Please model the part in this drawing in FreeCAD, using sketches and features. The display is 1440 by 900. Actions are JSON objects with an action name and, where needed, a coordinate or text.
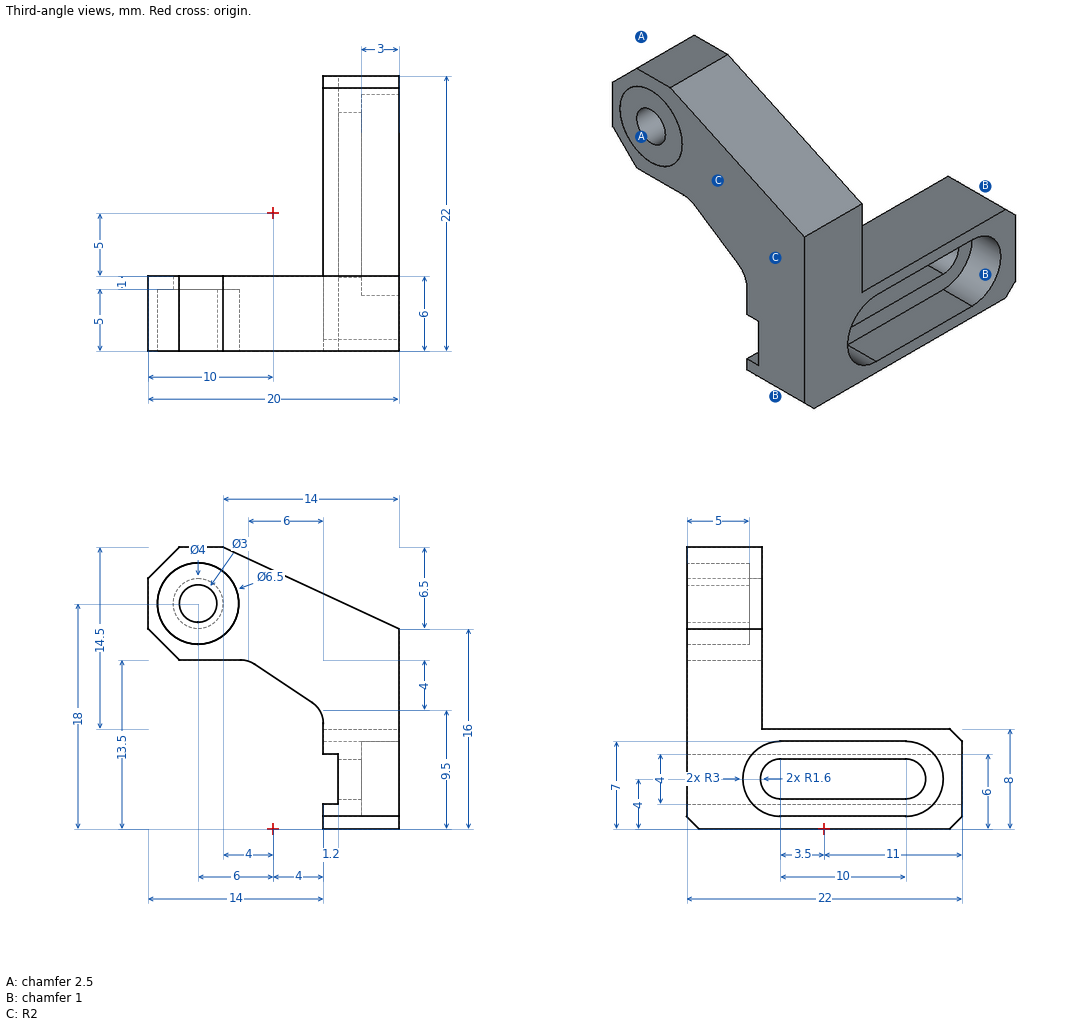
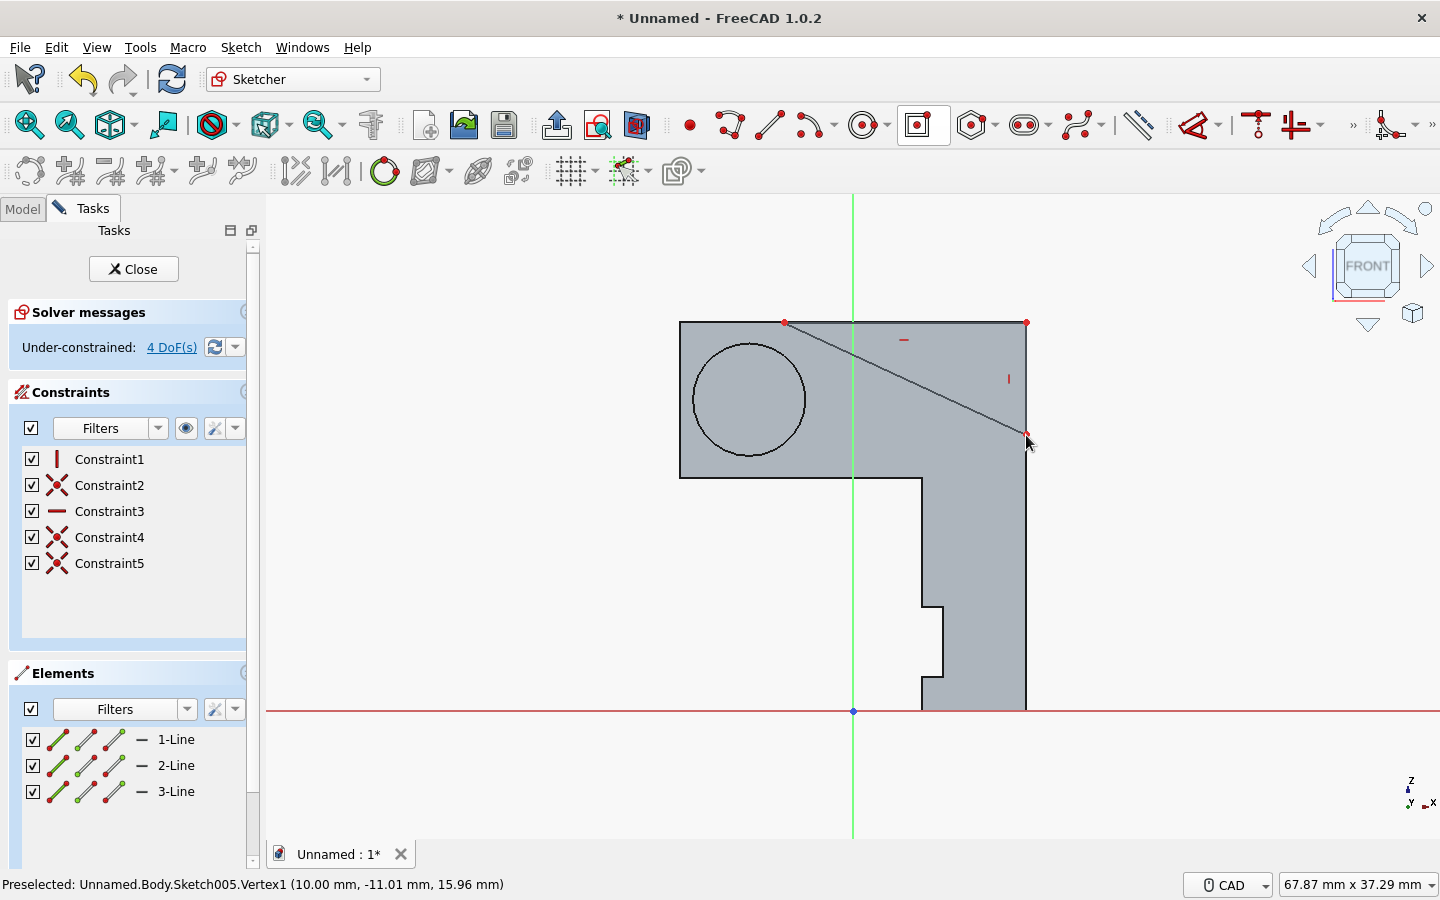
{"action": "left_click", "coordinate": [1194, 126]}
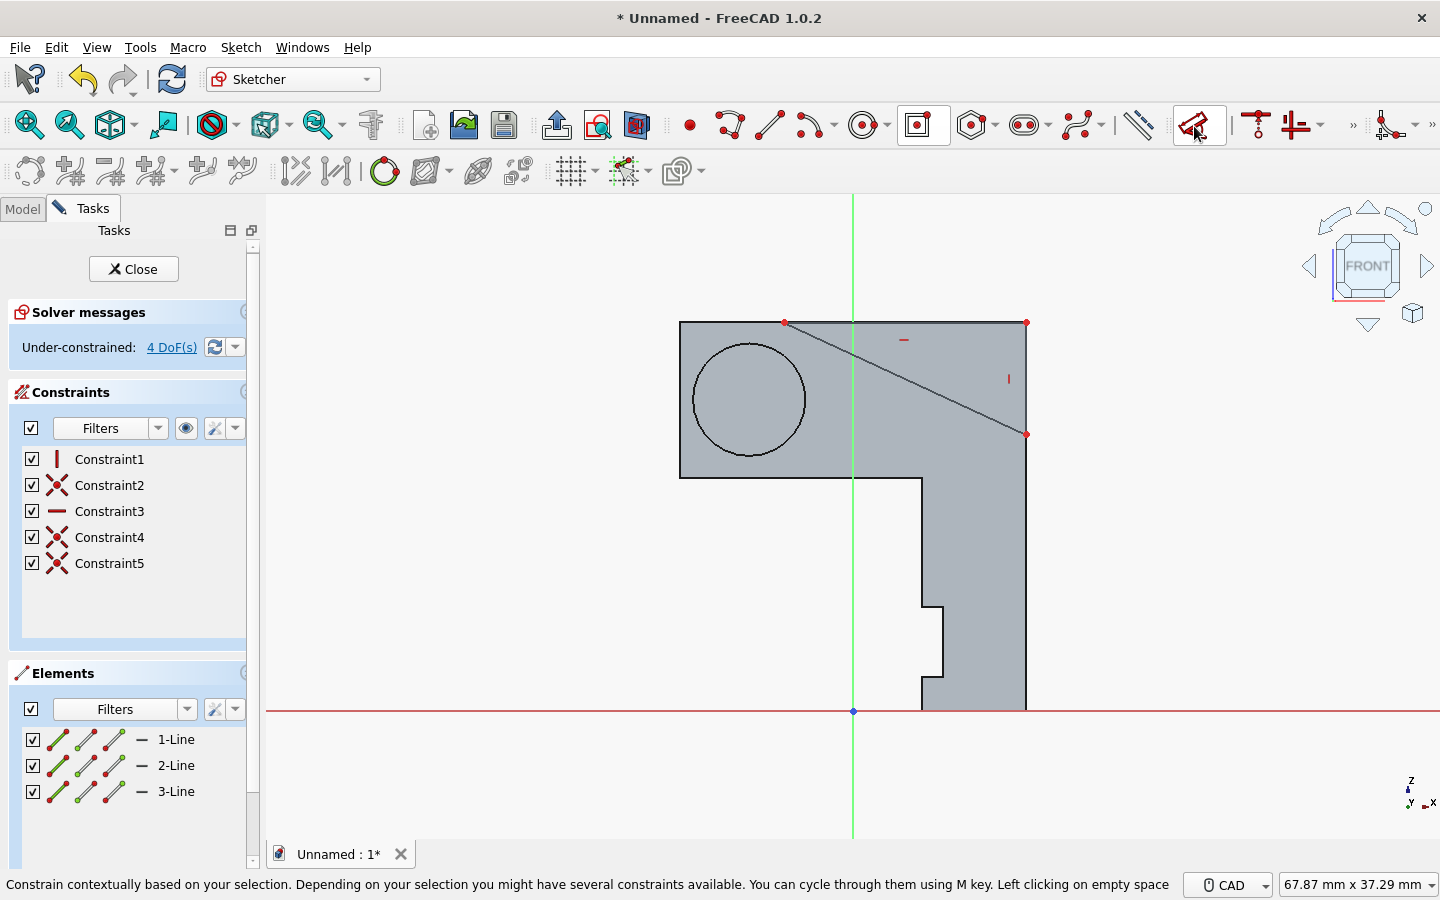
{"action": "left_click", "coordinate": [953, 323]}
{"action": "left_click", "coordinate": [905, 289]}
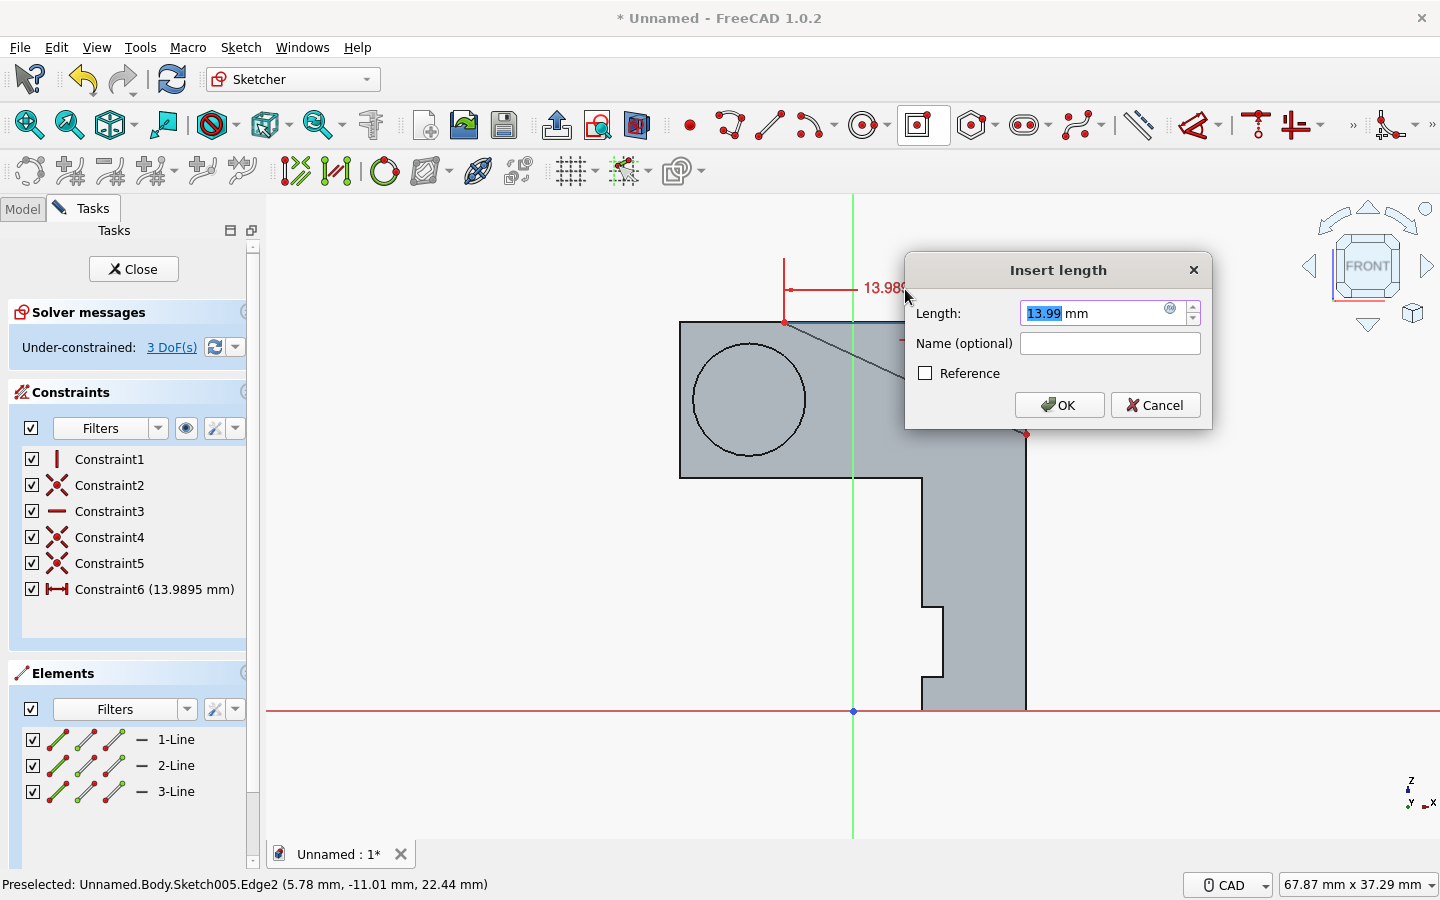
{"action": "type", "text": "14"}
{"action": "key", "text": "Return"}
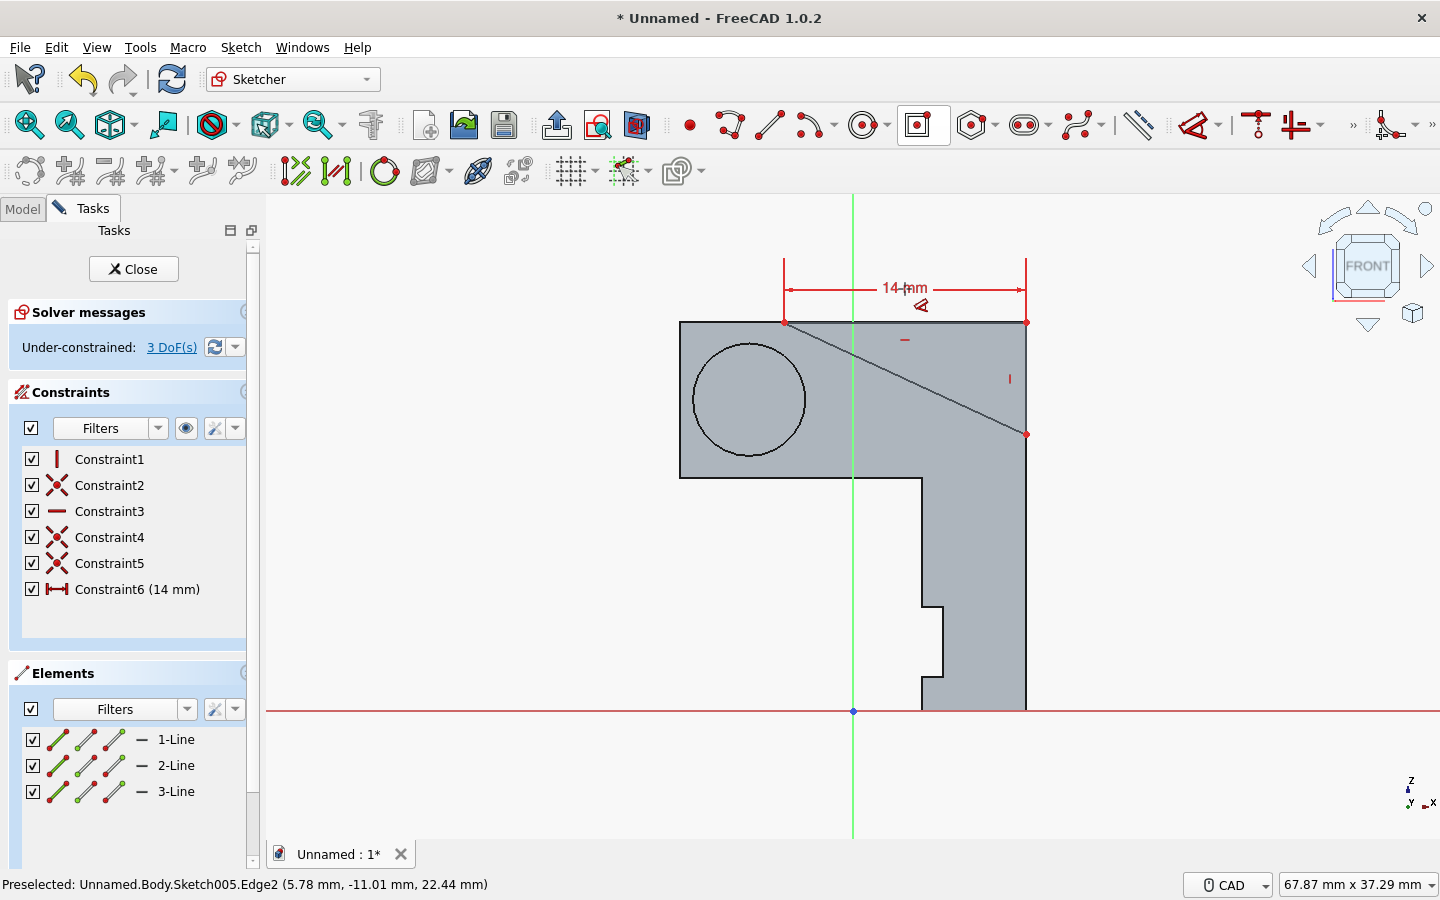
{"action": "left_click", "coordinate": [784, 323]}
{"action": "left_click", "coordinate": [818, 745]}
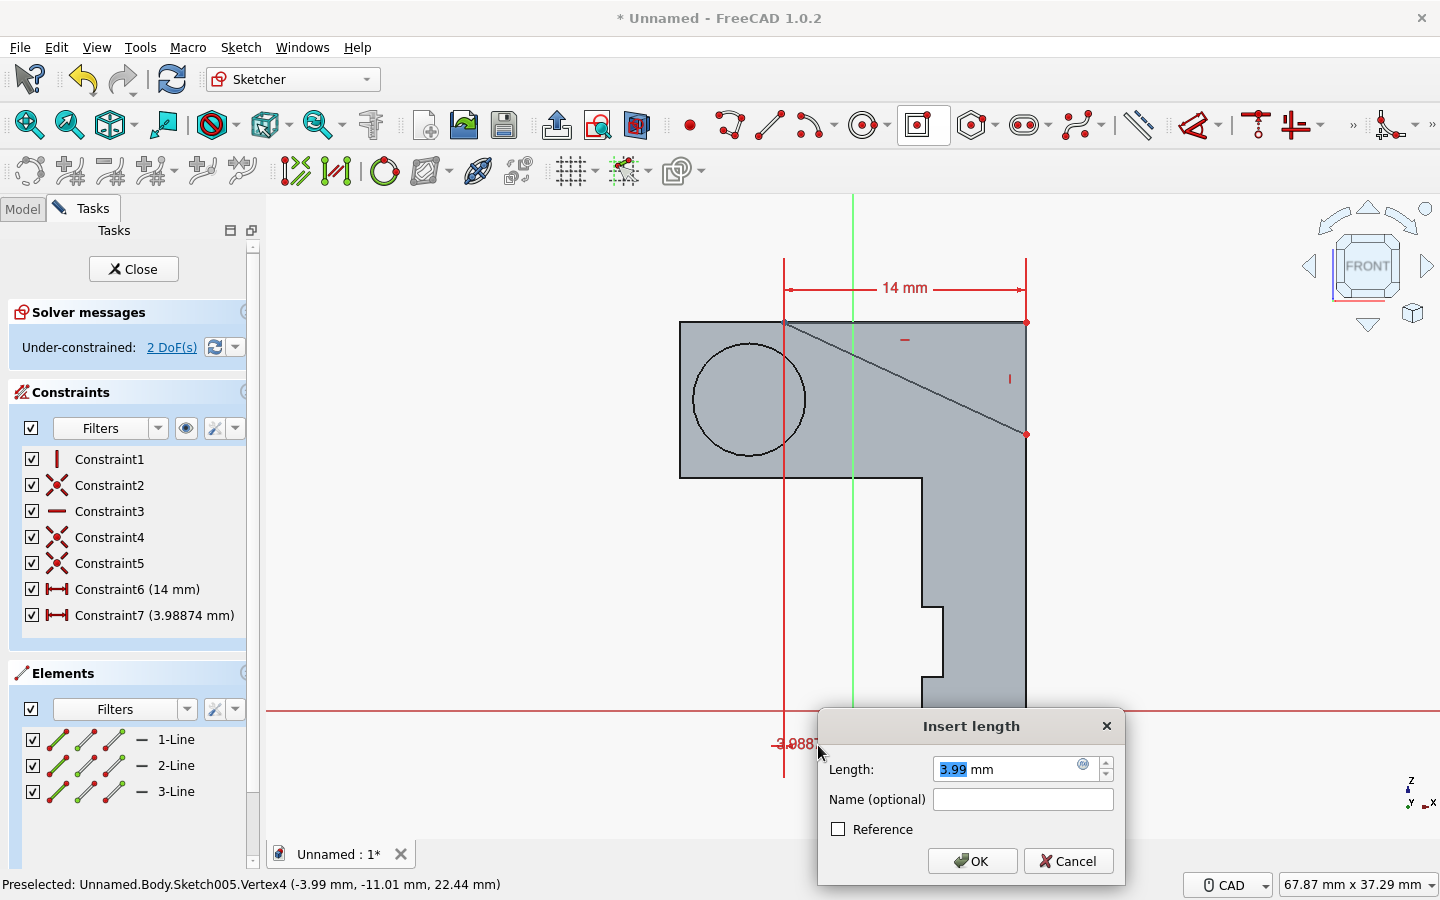
{"action": "type", "text": "4"}
{"action": "key", "text": "Return"}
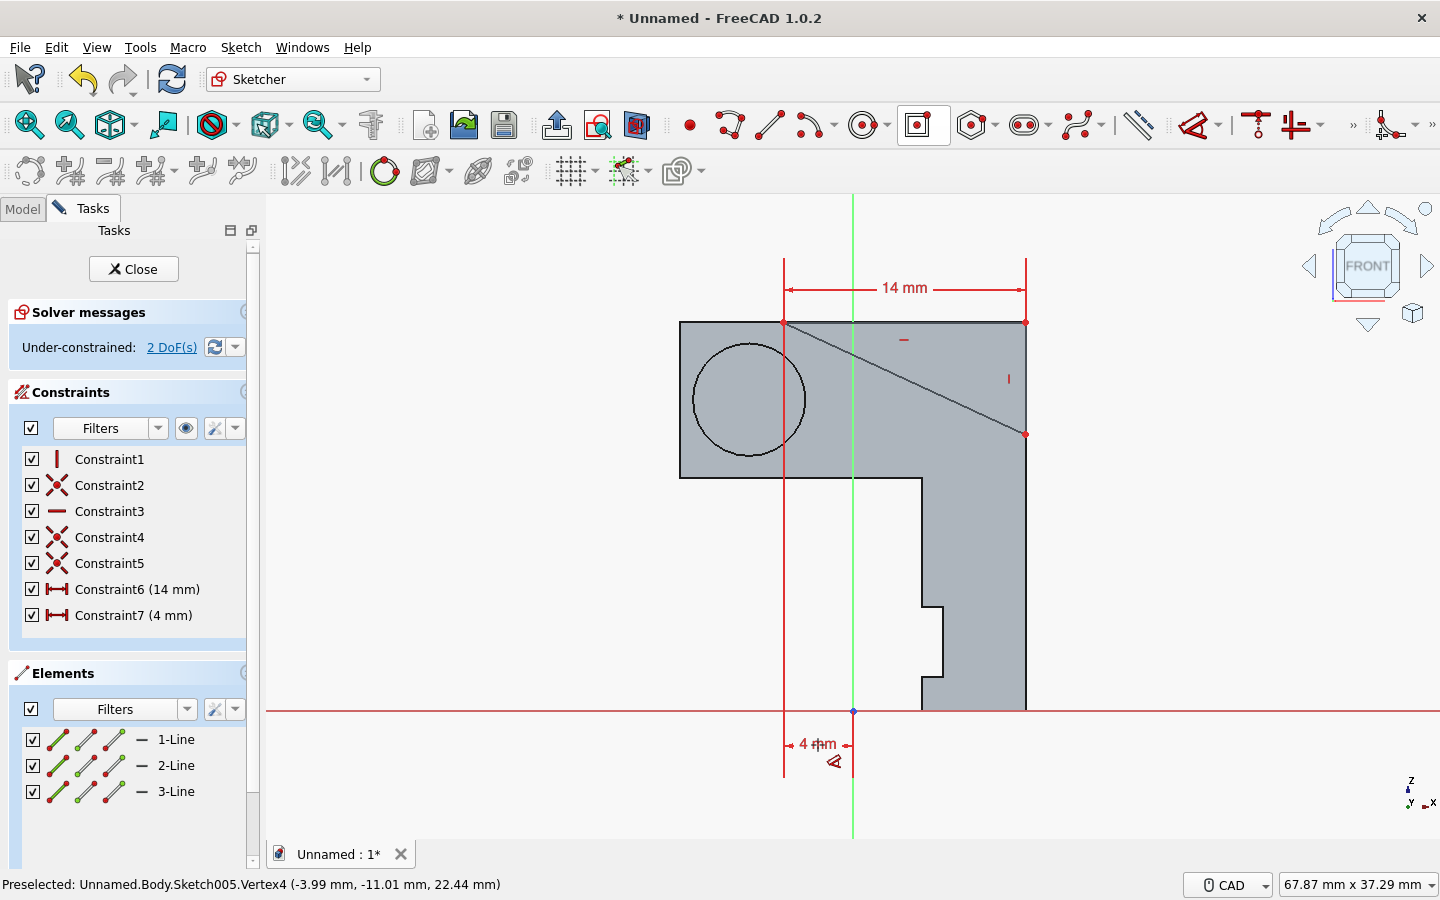
{"action": "left_click", "coordinate": [1026, 401]}
{"action": "left_click", "coordinate": [1060, 379]}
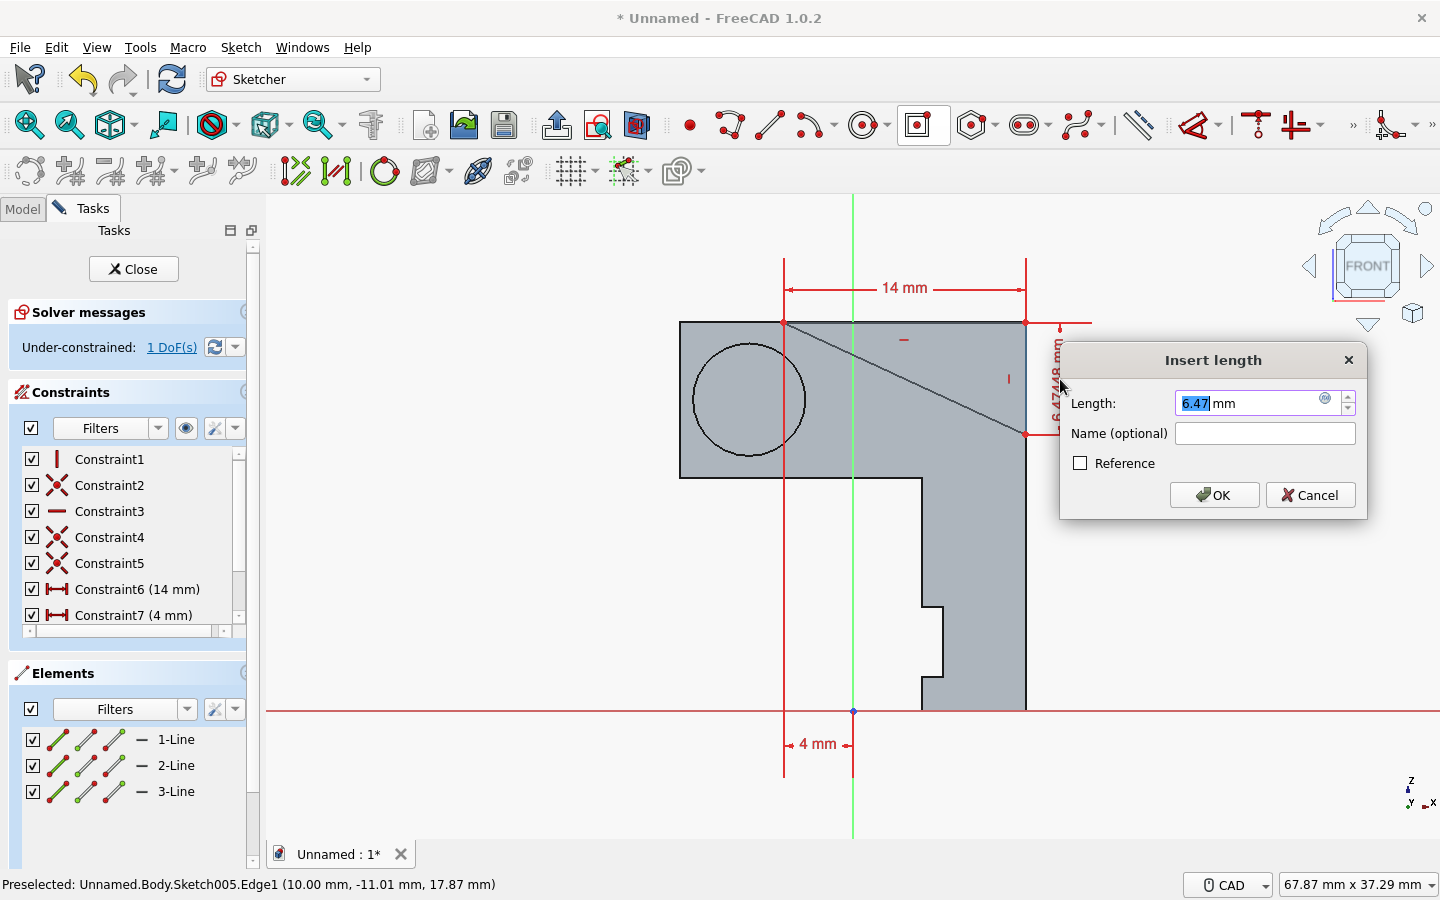
{"action": "type", "text": "6.5"}
{"action": "key", "text": "Return"}